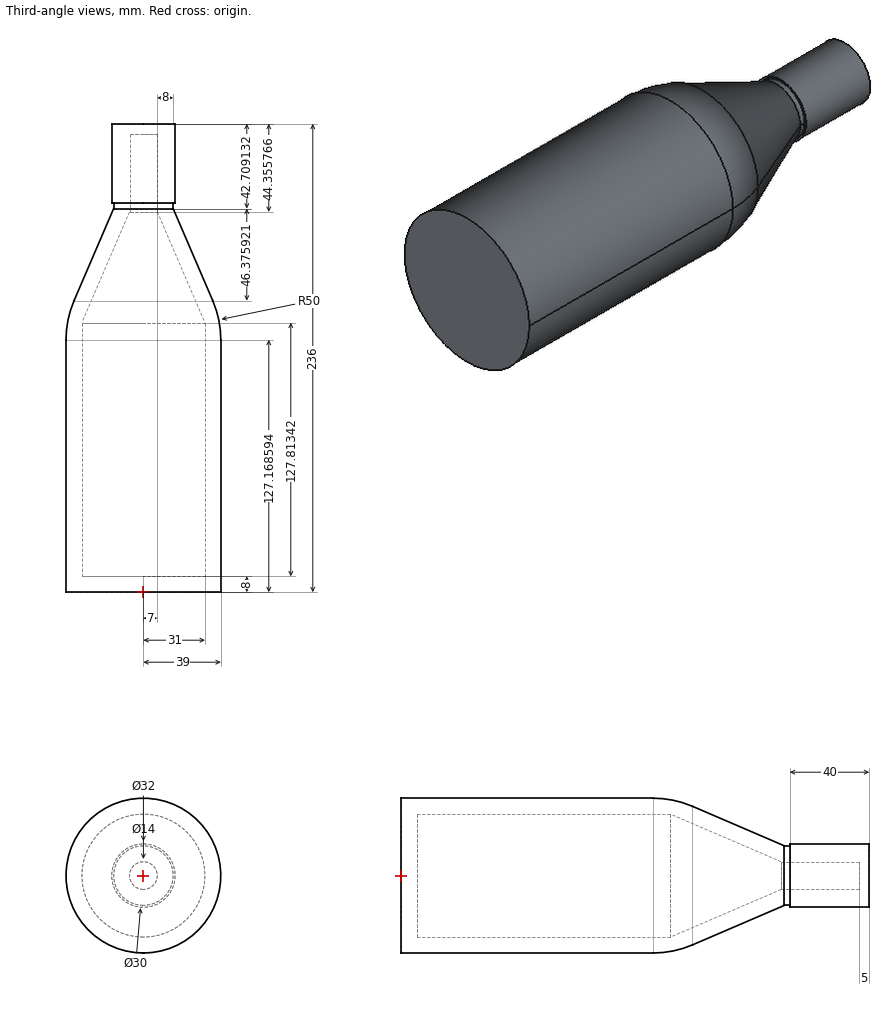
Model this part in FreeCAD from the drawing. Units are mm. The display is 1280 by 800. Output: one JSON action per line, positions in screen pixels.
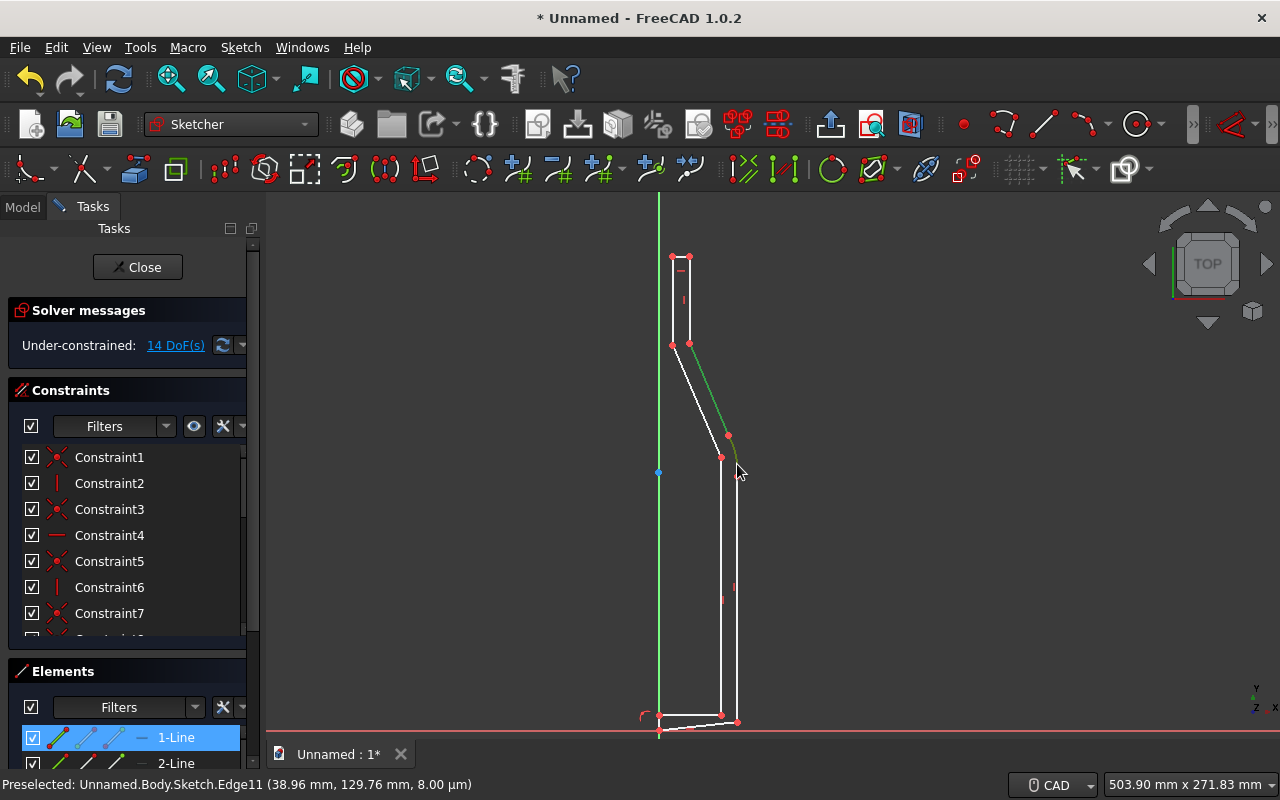
{"action": "key", "text": "t"}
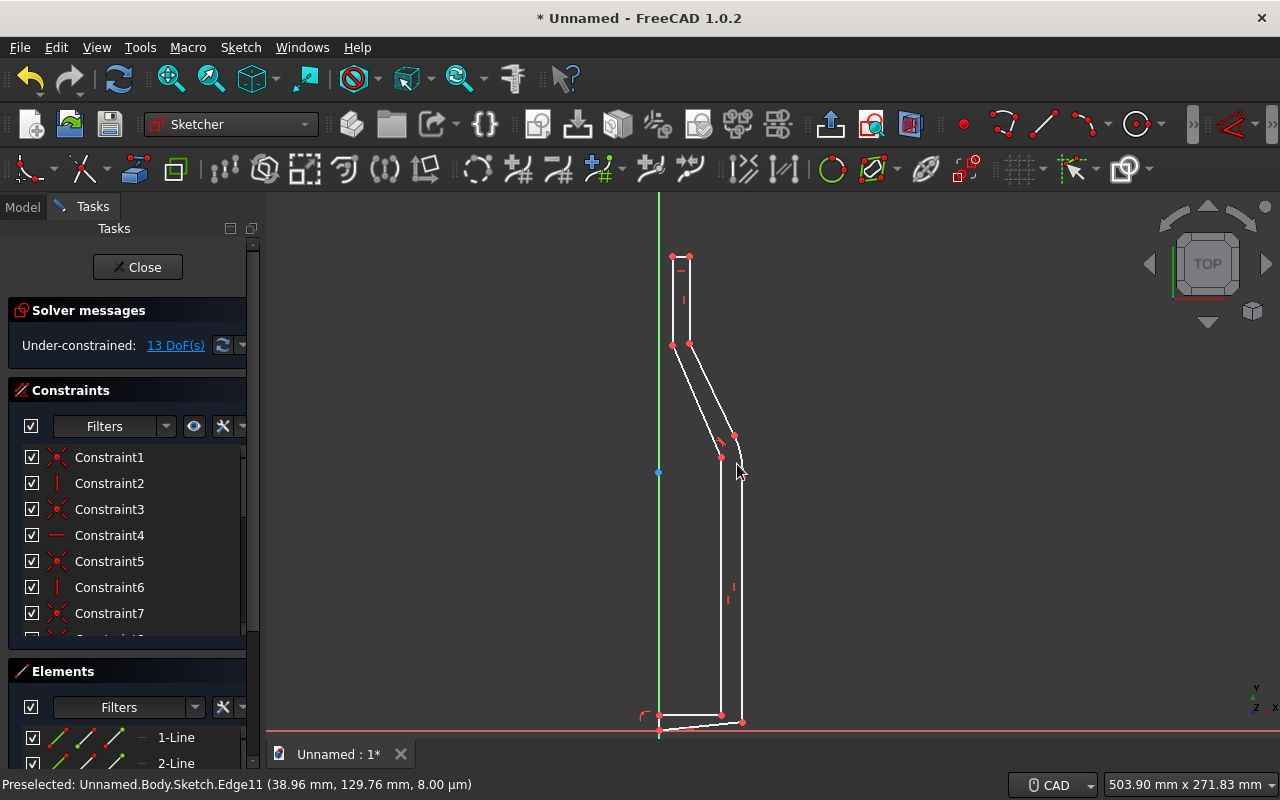
{"action": "scroll", "coordinate": [717, 409], "scroll_direction": "down", "scroll_amount": 2}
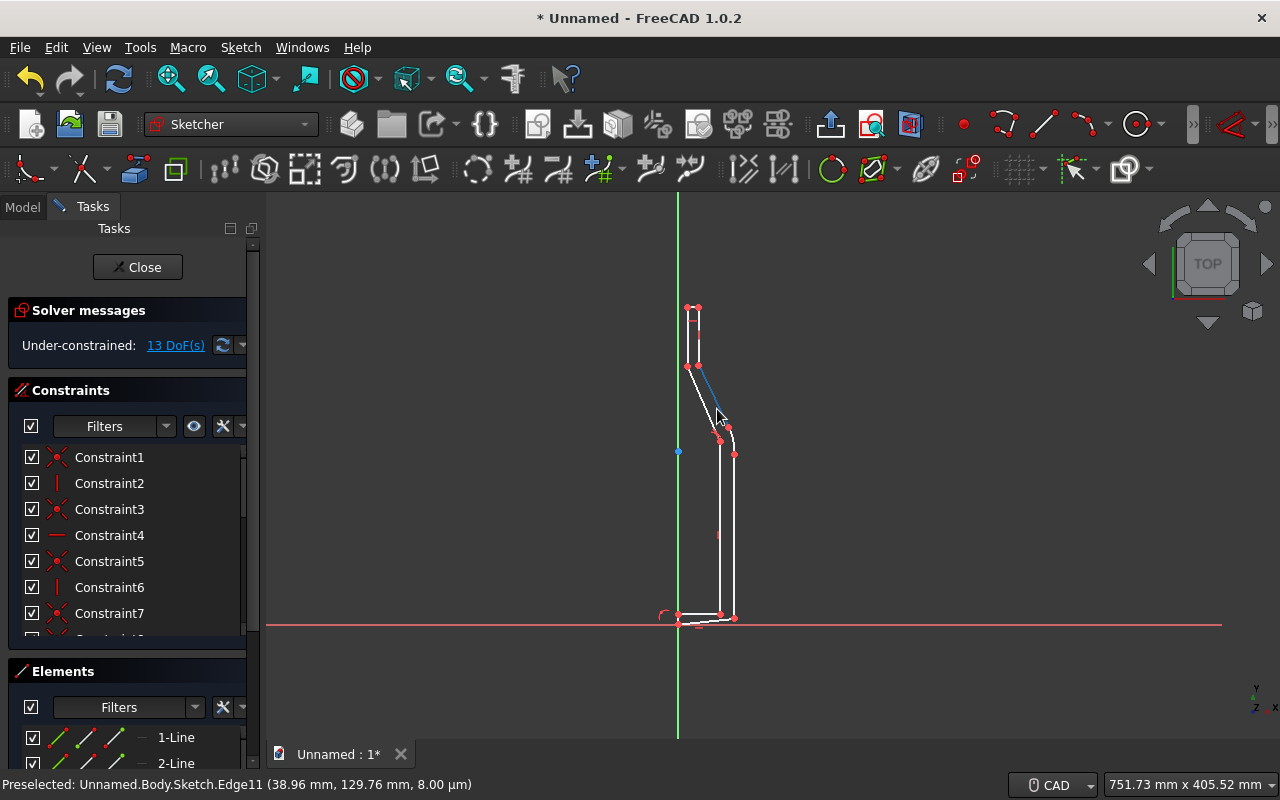
{"action": "scroll", "coordinate": [695, 623], "scroll_direction": "up", "scroll_amount": 3}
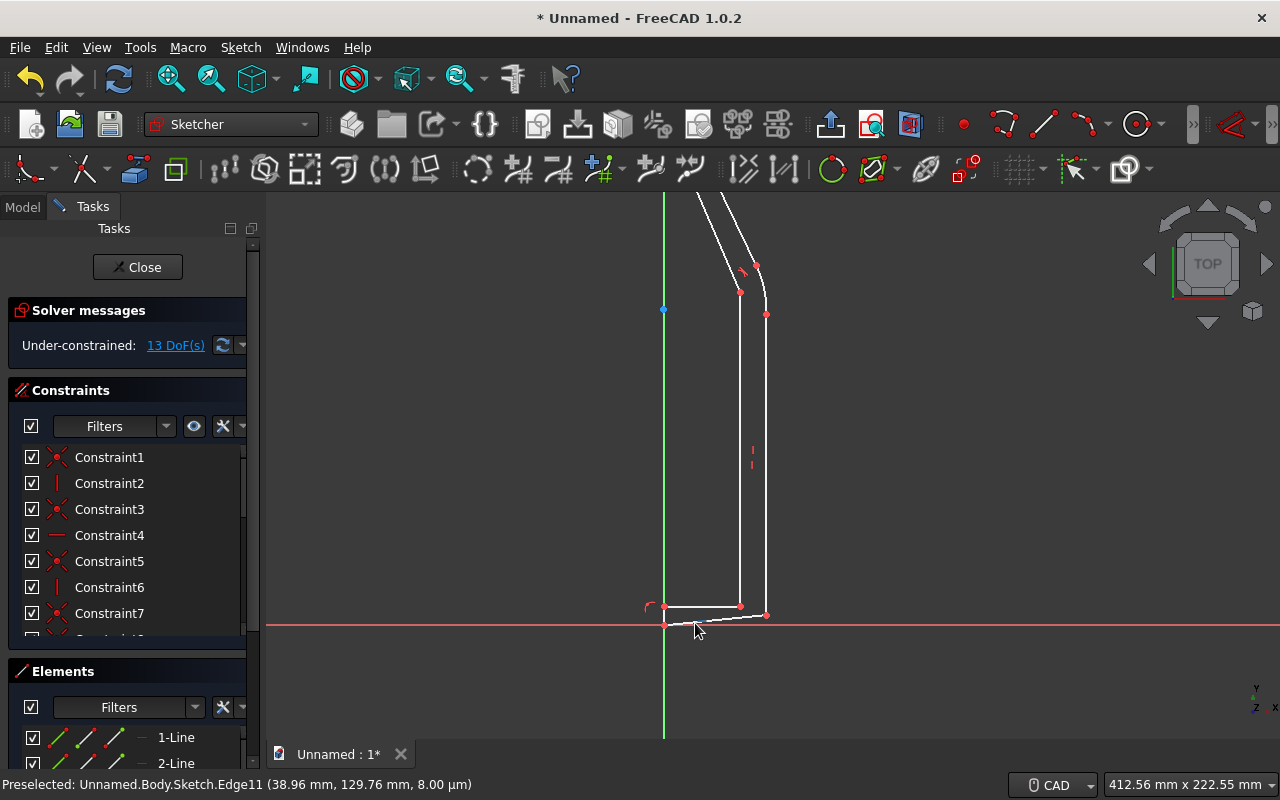
{"action": "left_click", "coordinate": [695, 622]}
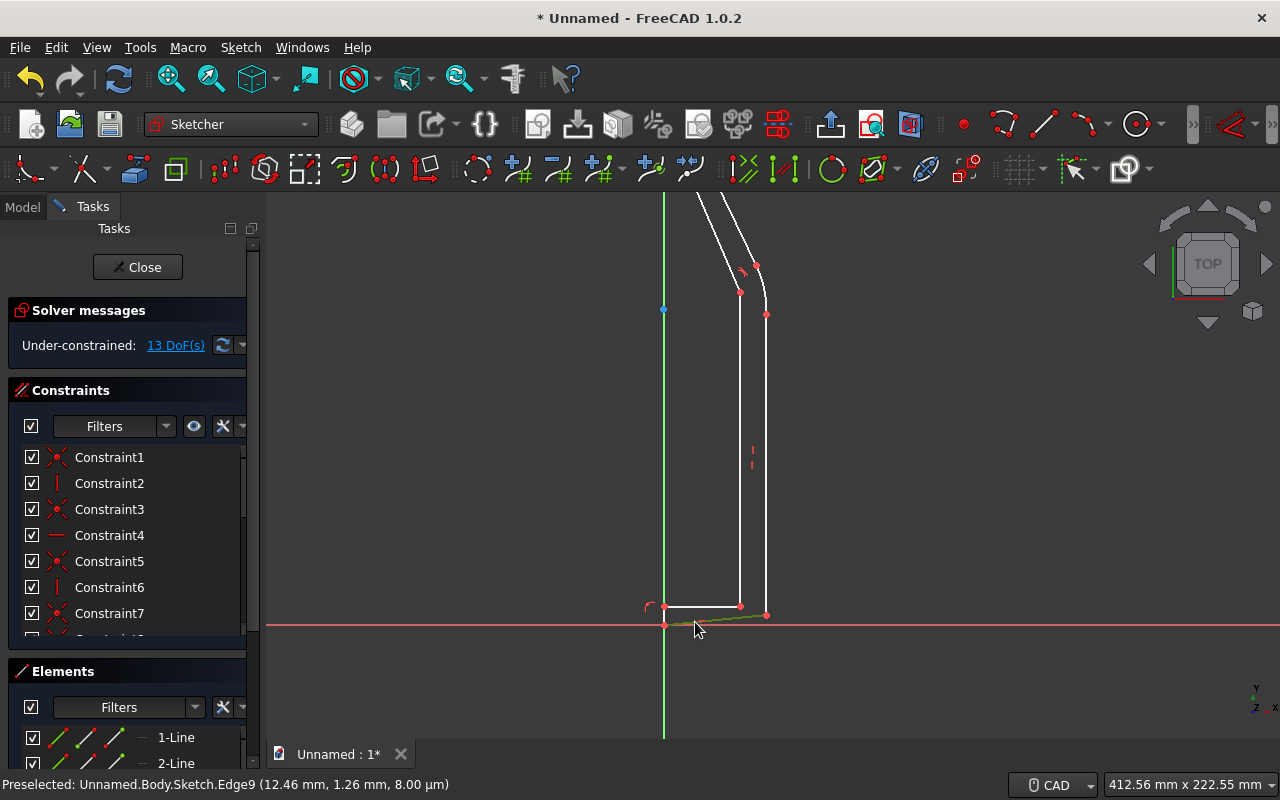
{"action": "key", "text": "h"}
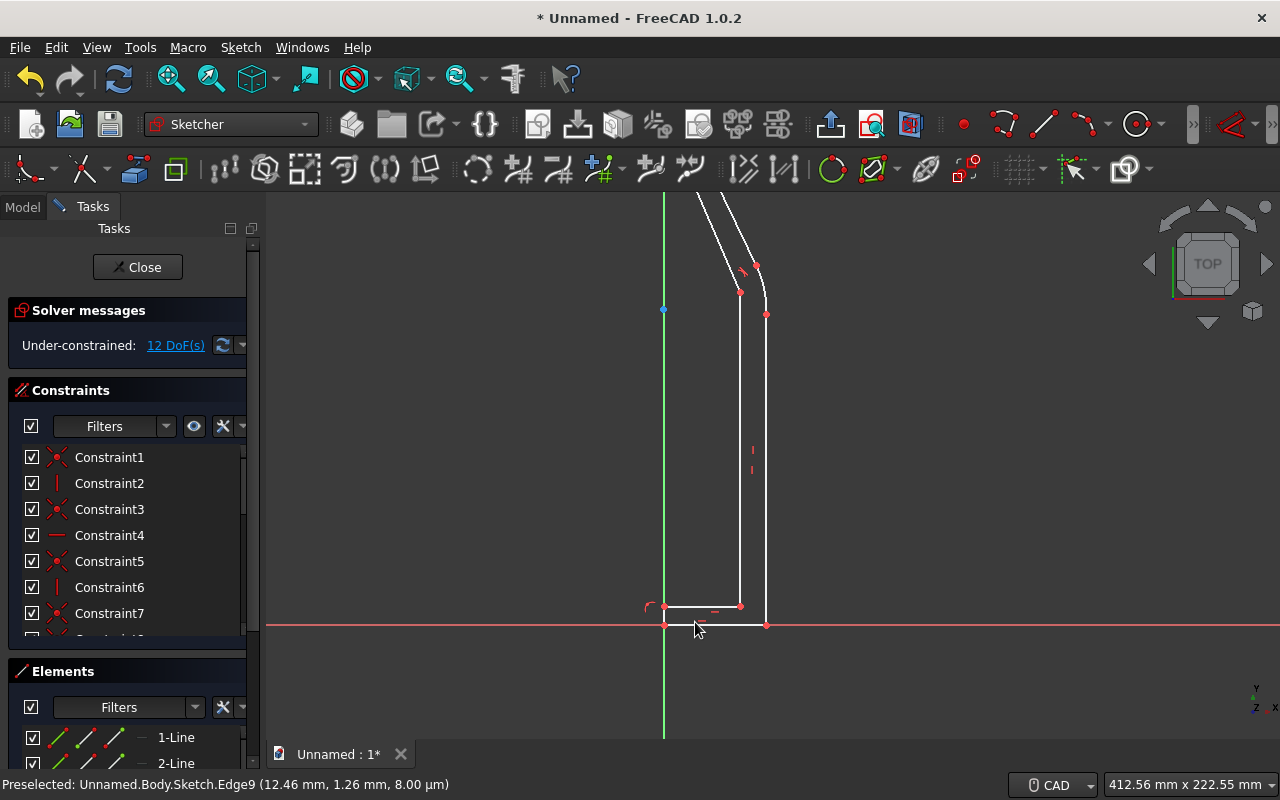
{"action": "left_click", "coordinate": [1232, 124]}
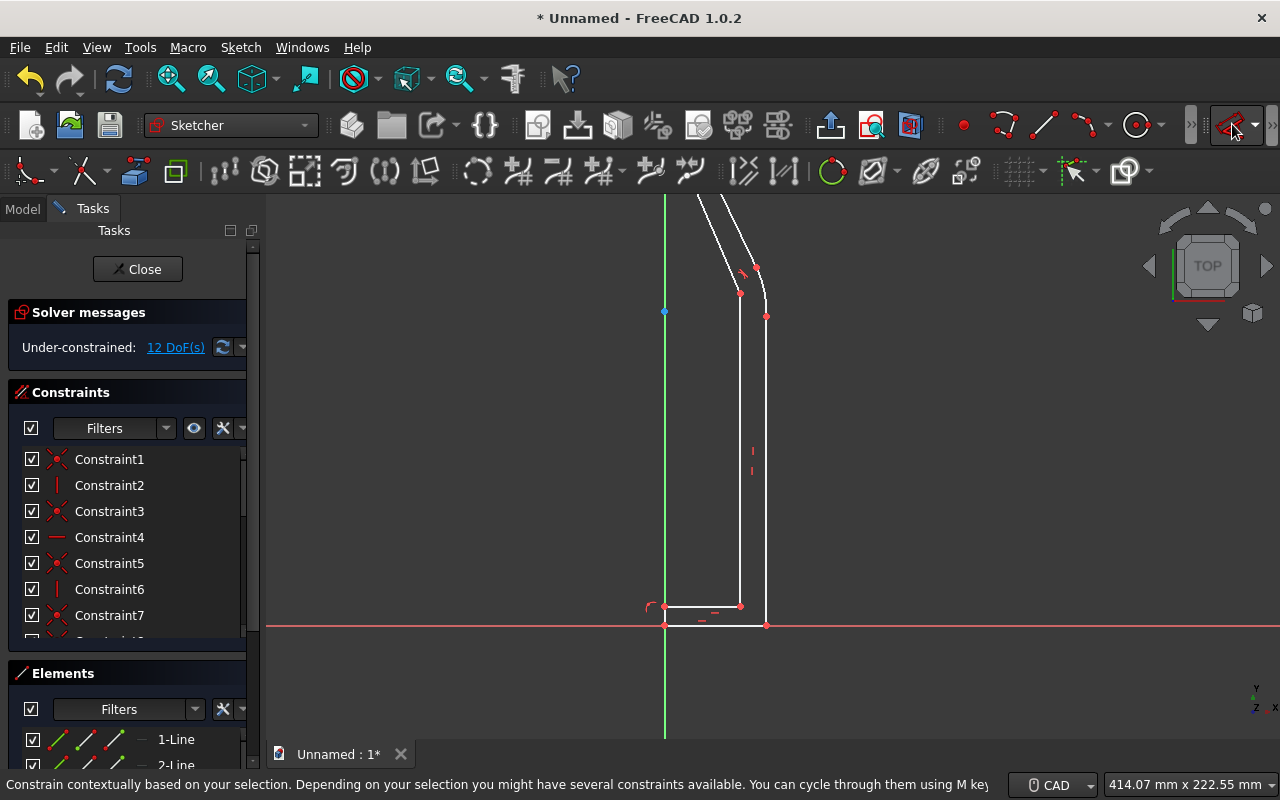
{"action": "left_click", "coordinate": [766, 301]}
{"action": "left_click", "coordinate": [798, 298]}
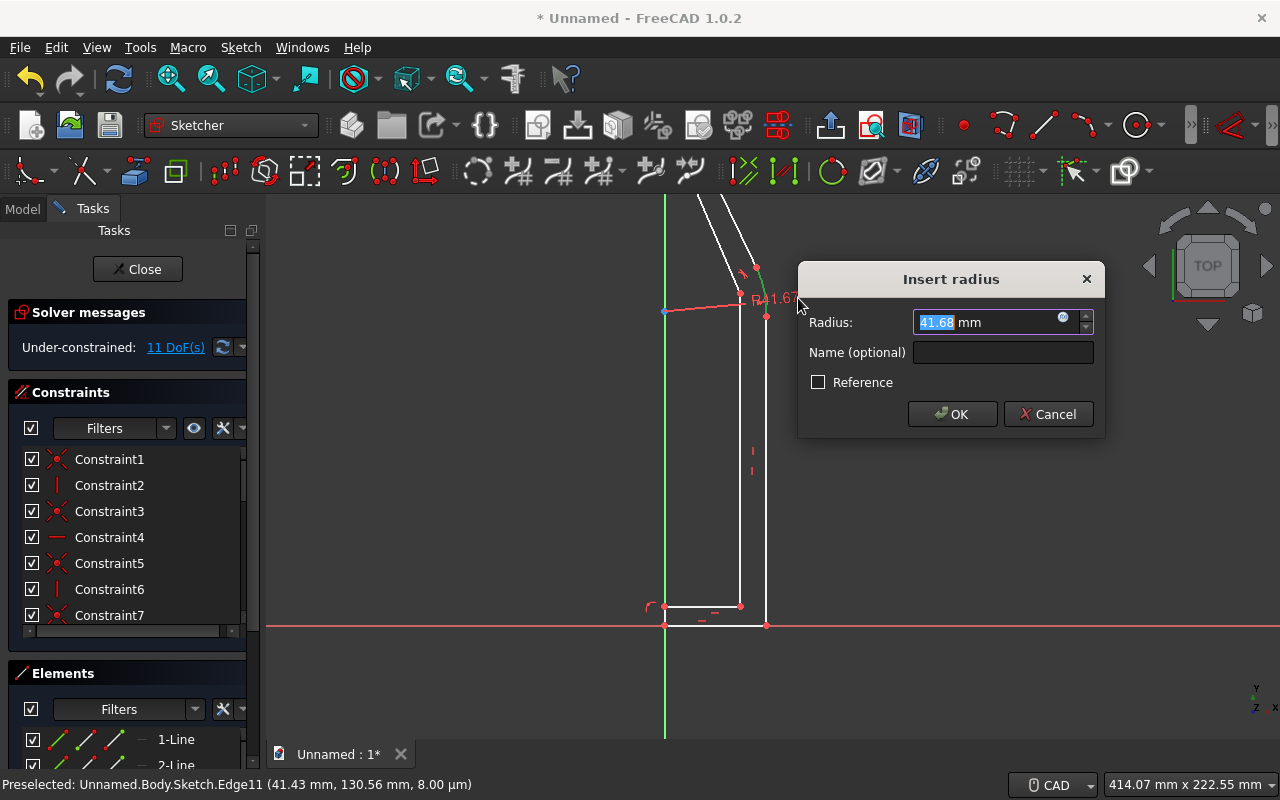
{"action": "type", "text": "50"}
{"action": "key", "text": "Return"}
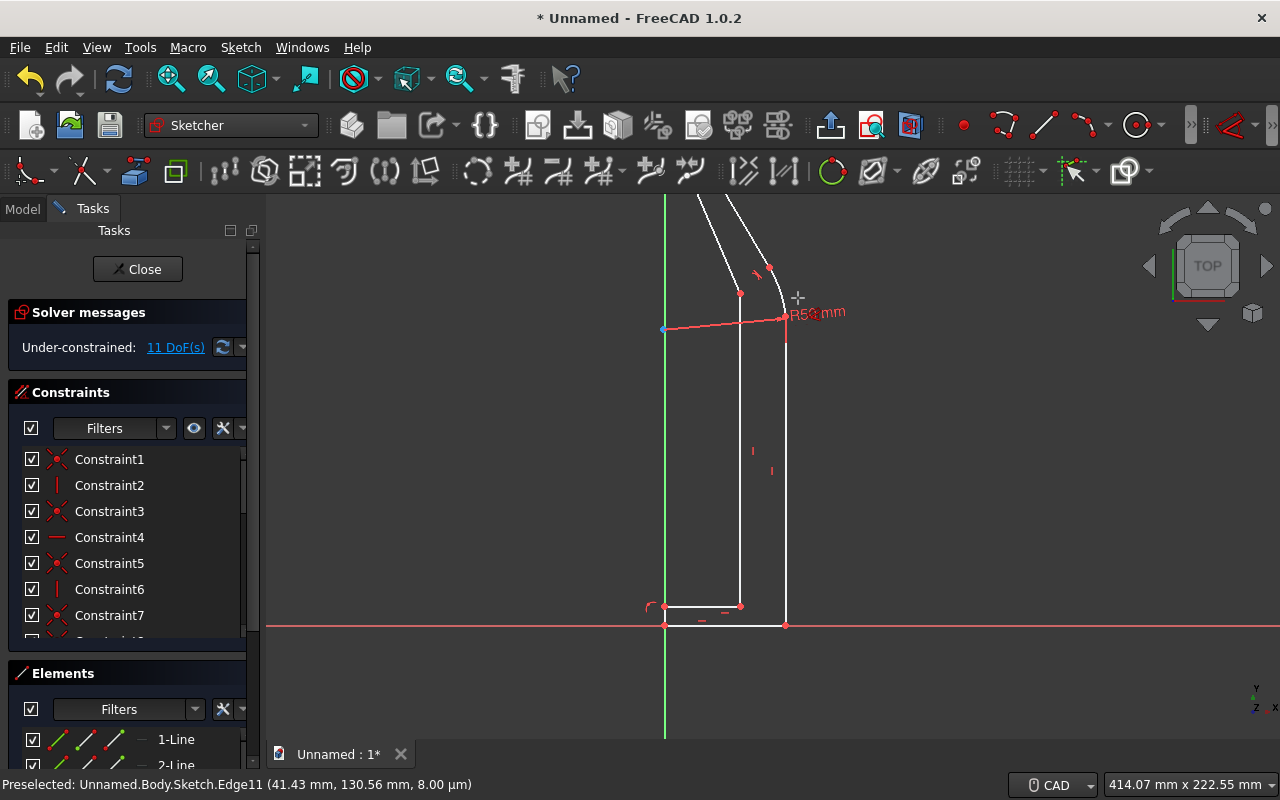
{"action": "scroll", "coordinate": [695, 624], "scroll_direction": "down", "scroll_amount": 3}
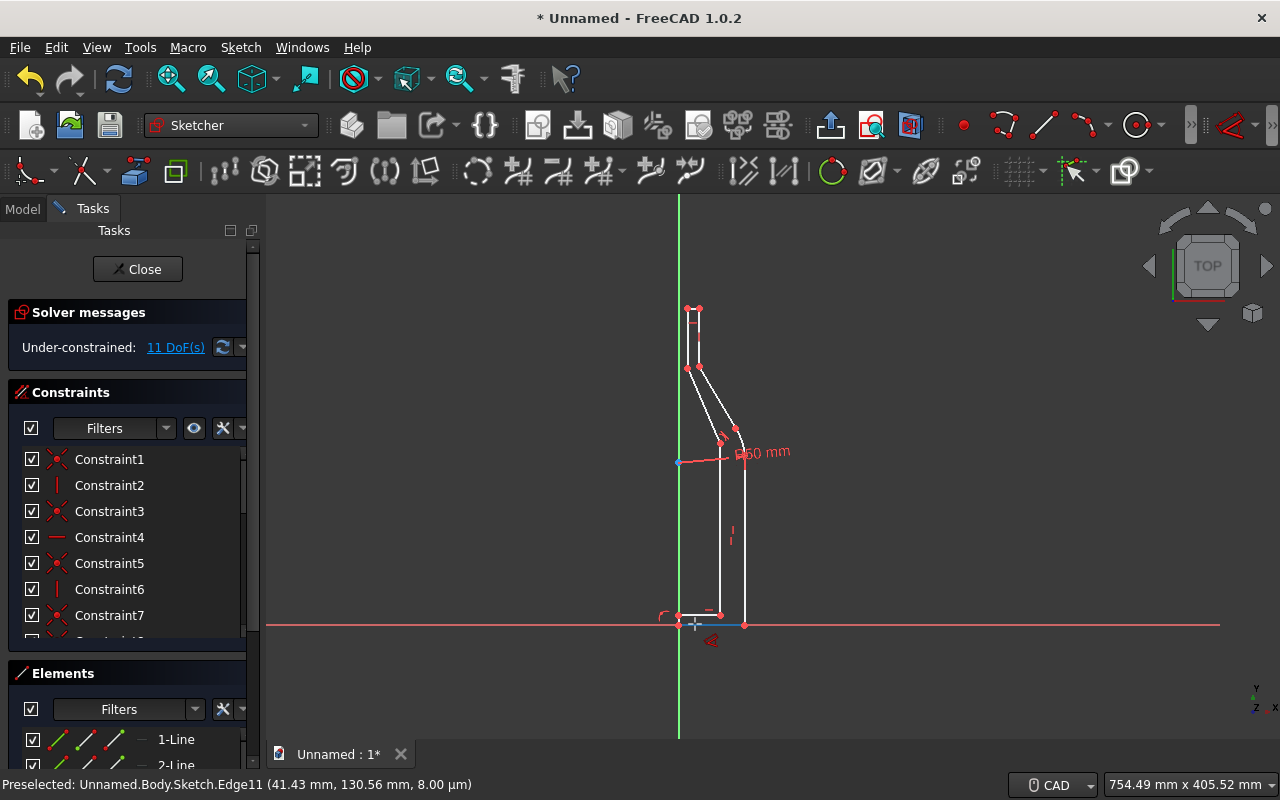
{"action": "scroll", "coordinate": [693, 309], "scroll_direction": "up", "scroll_amount": 7}